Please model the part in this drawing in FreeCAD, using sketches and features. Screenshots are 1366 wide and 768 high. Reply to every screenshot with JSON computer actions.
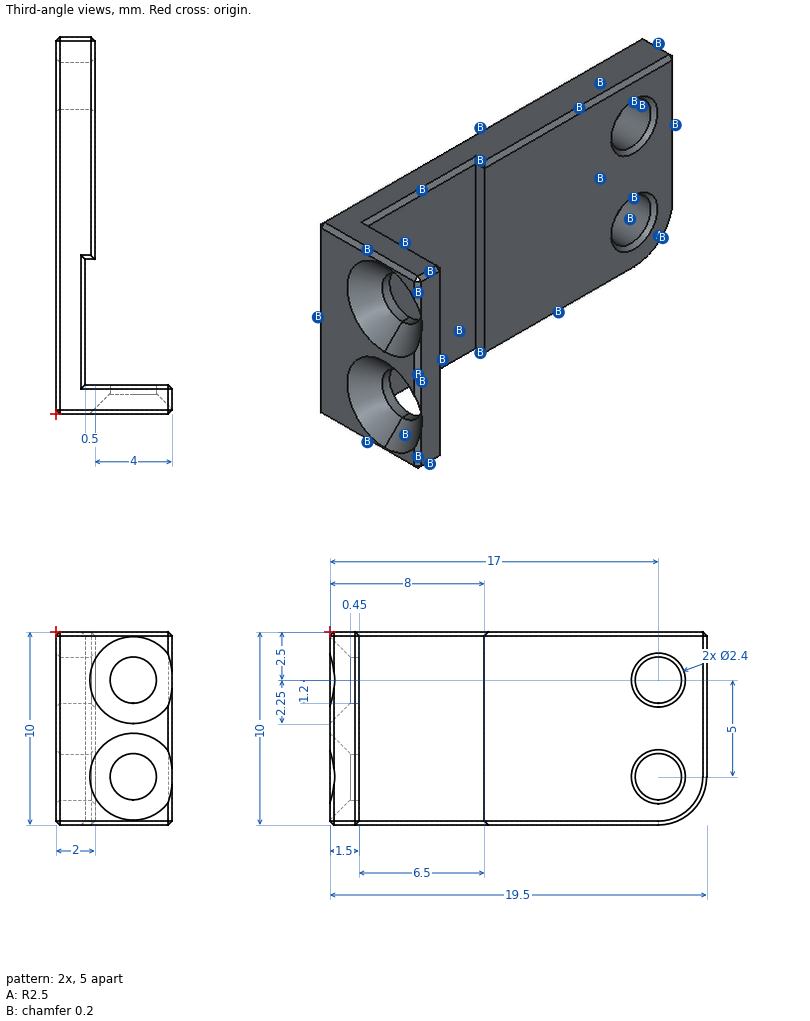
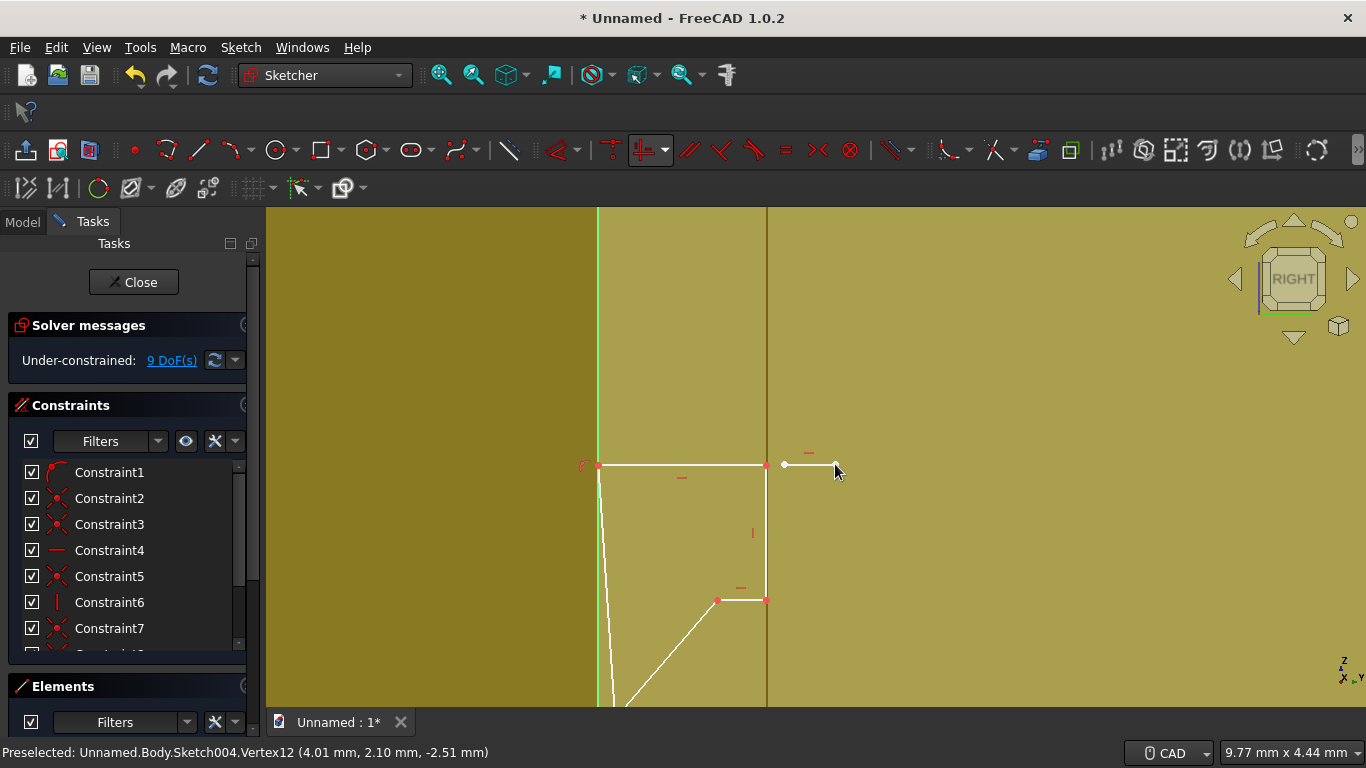
{"action": "left_click", "coordinate": [799, 465]}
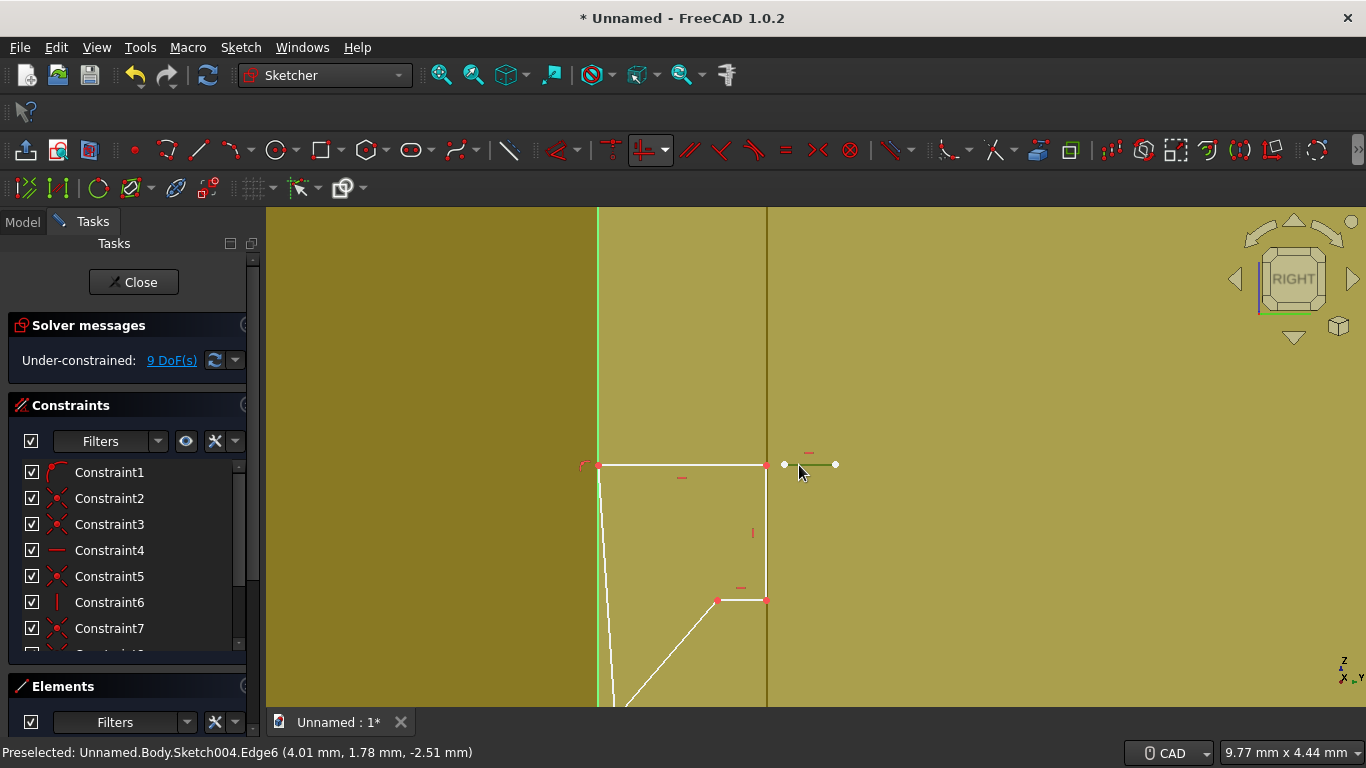
{"action": "left_click", "coordinate": [510, 150]}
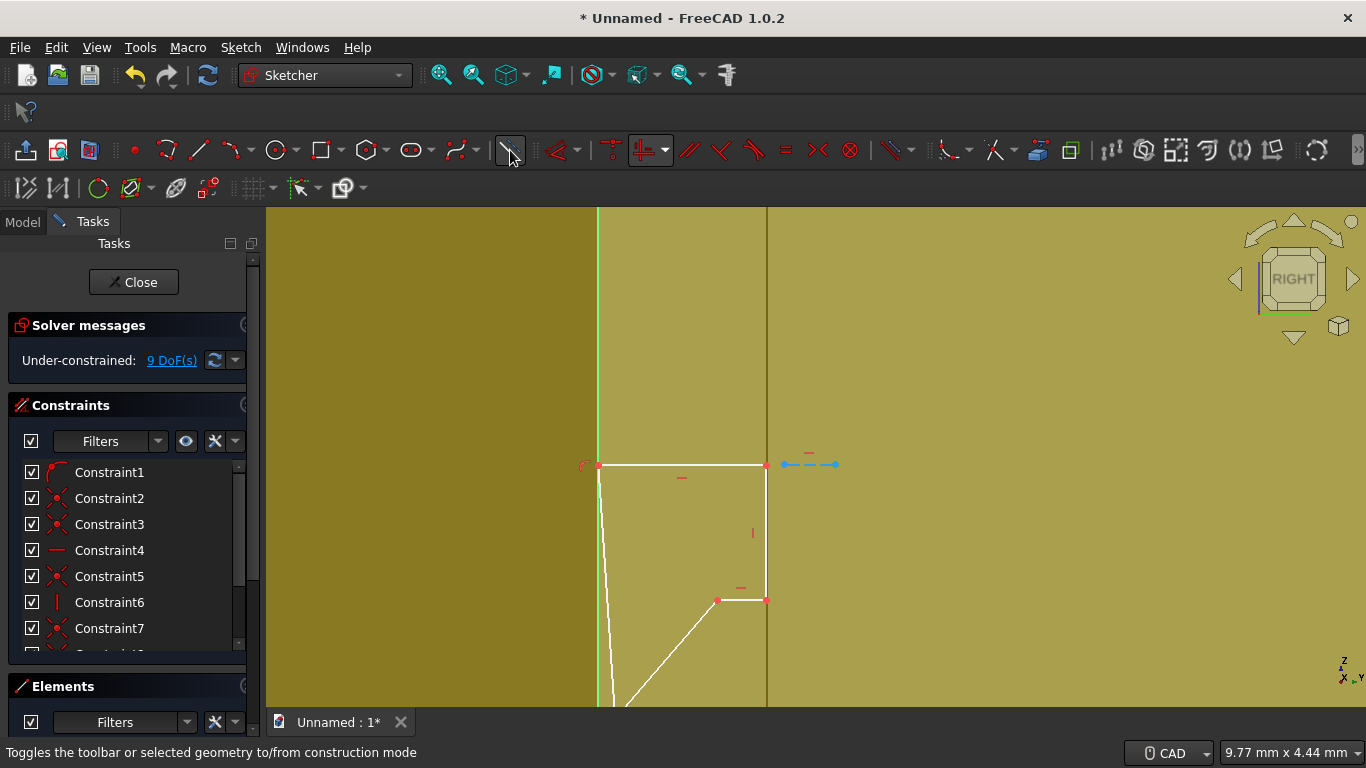
{"action": "left_click", "coordinate": [610, 643]}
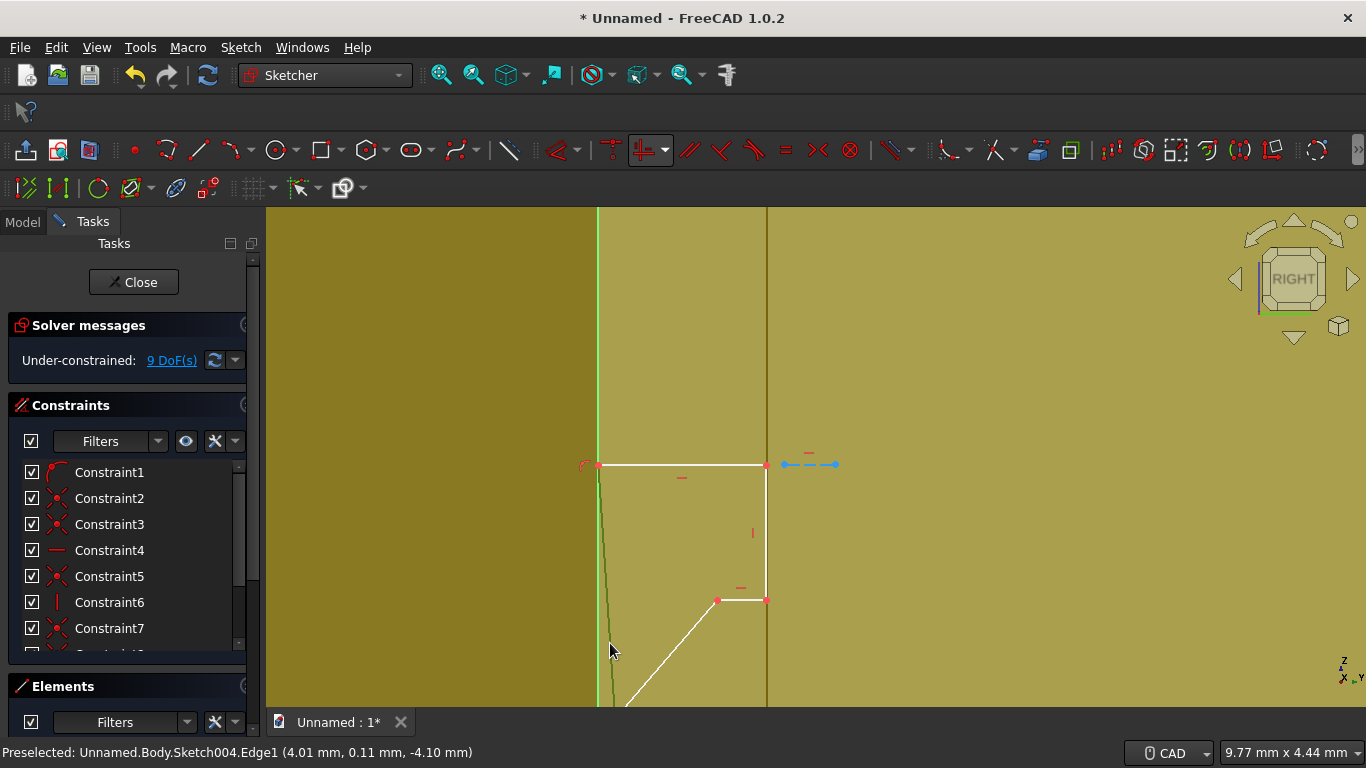
{"action": "left_click", "coordinate": [668, 150]}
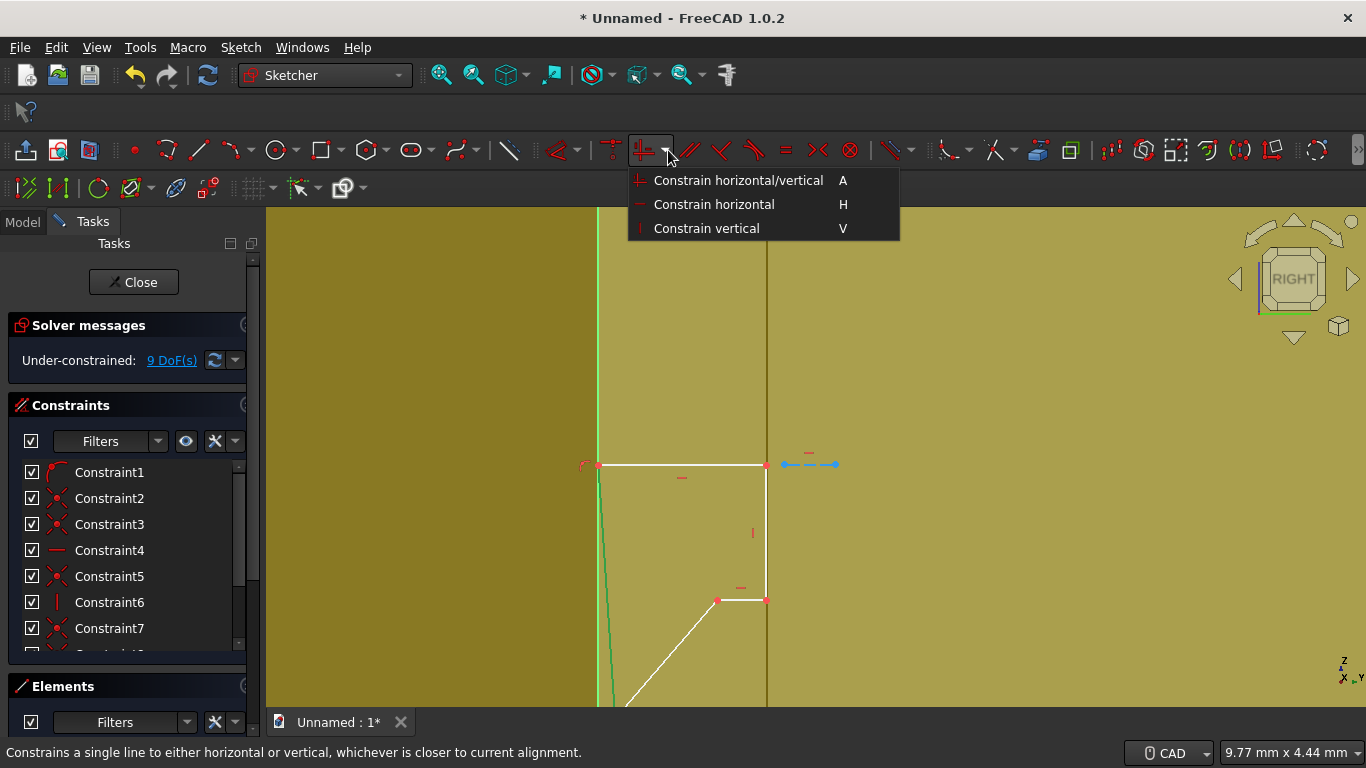
{"action": "left_click", "coordinate": [764, 228]}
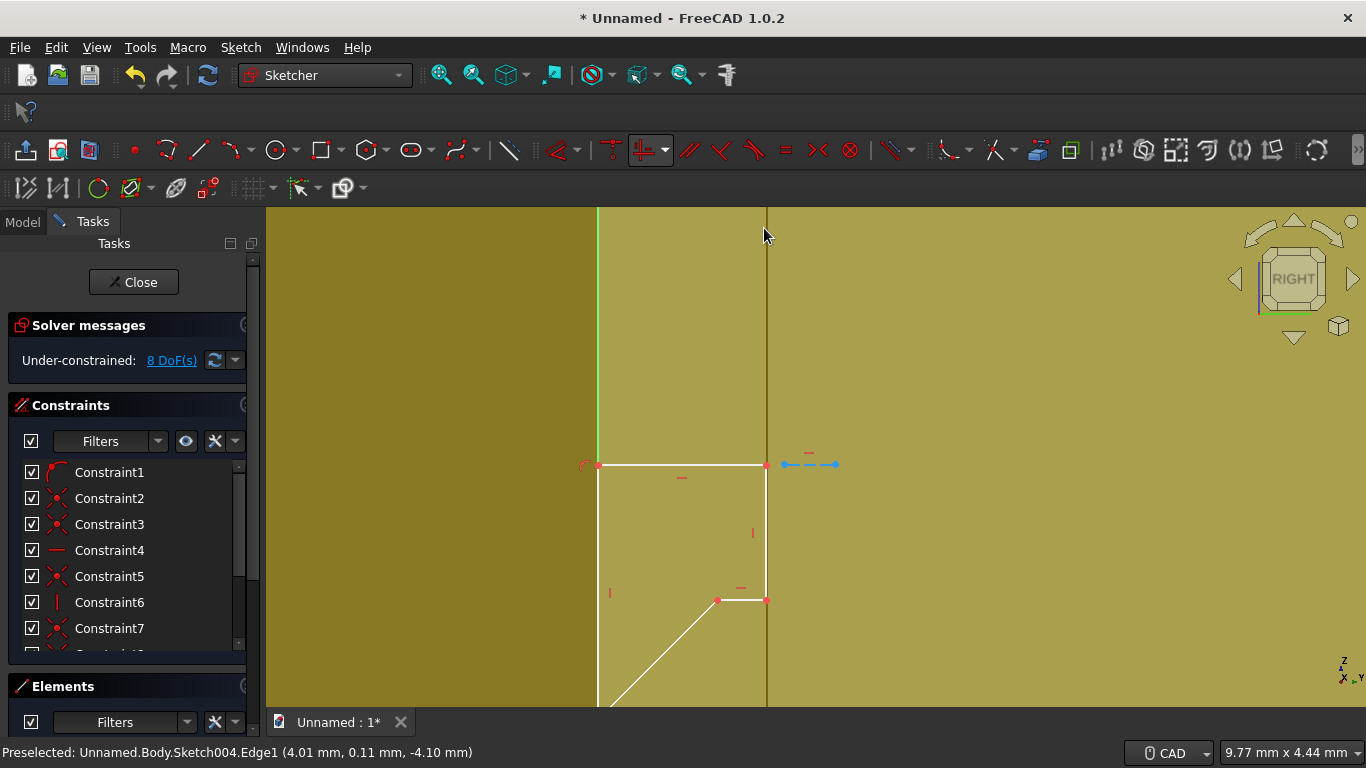
{"action": "left_click", "coordinate": [556, 150]}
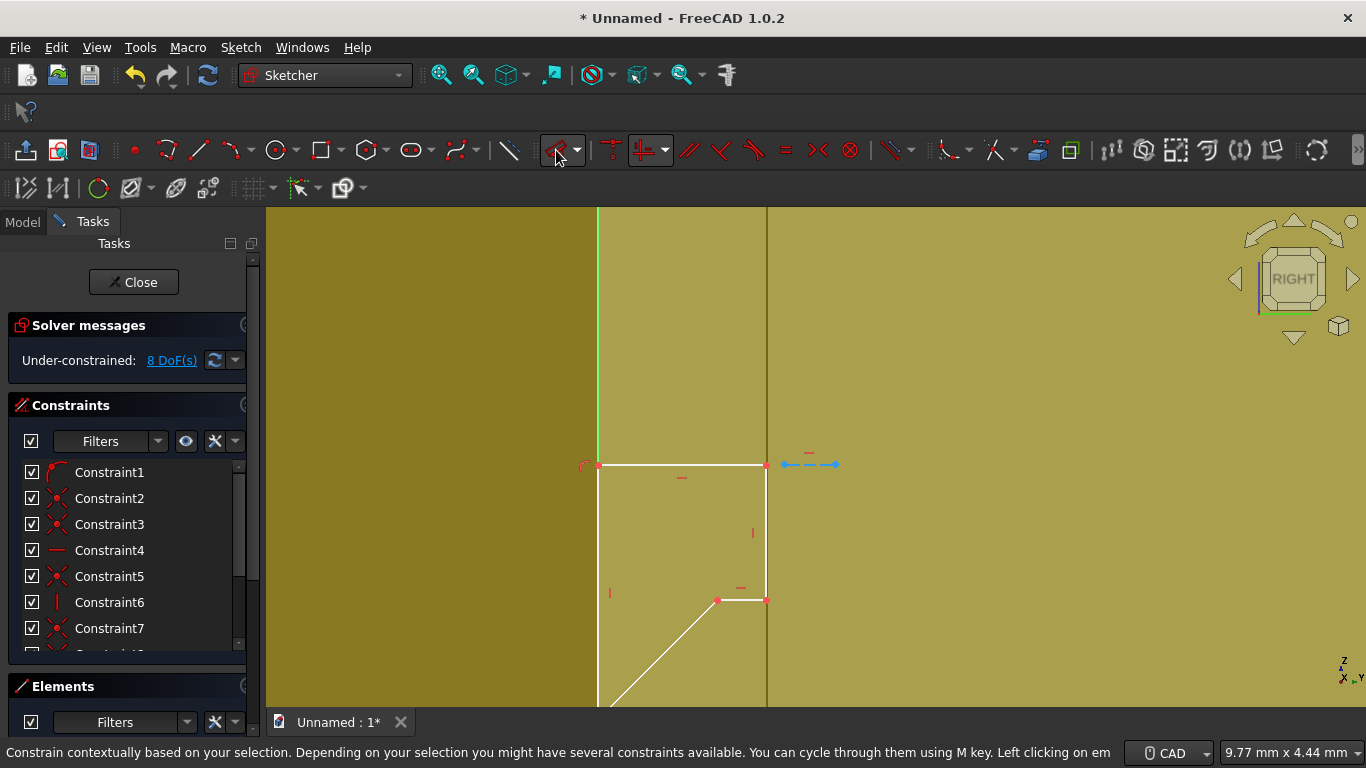
{"action": "left_click", "coordinate": [766, 560]}
{"action": "left_click", "coordinate": [800, 533]}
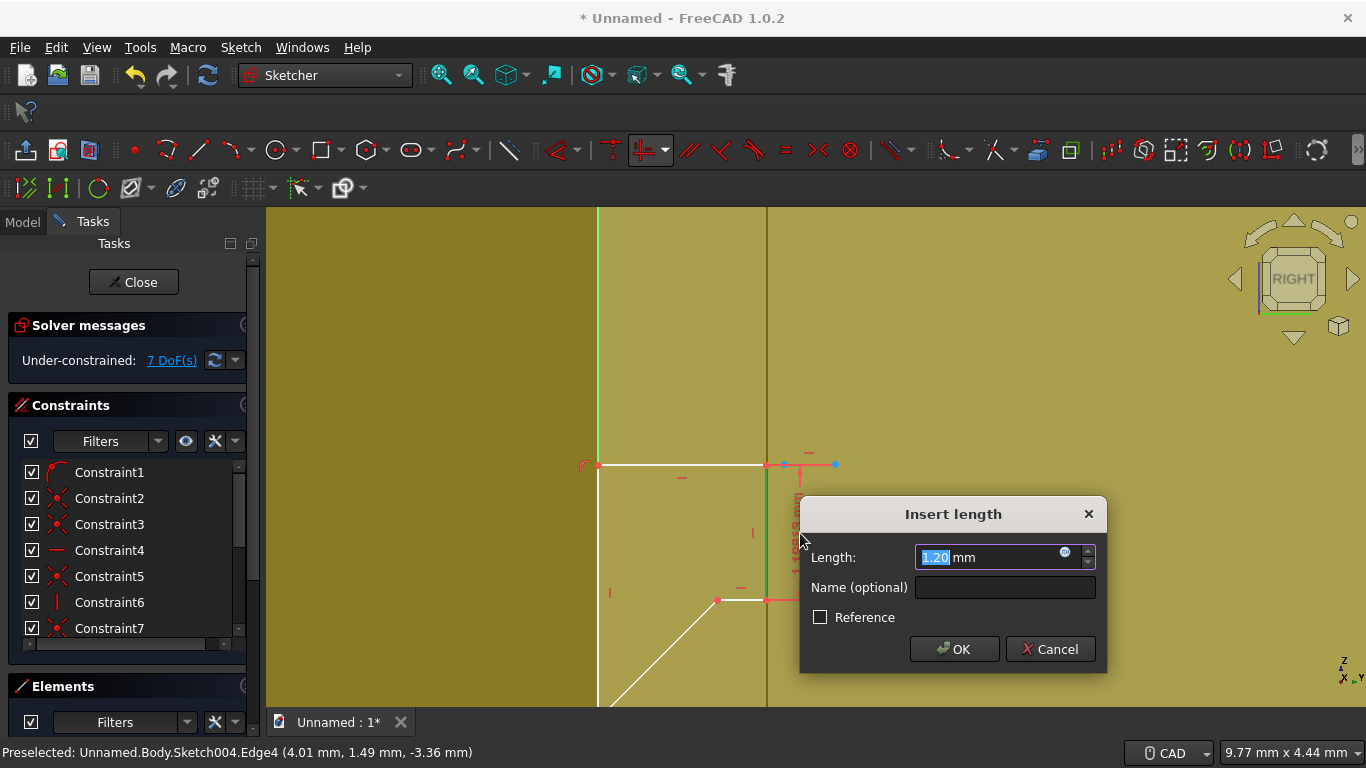
{"action": "type", "text": "1.2"}
{"action": "key", "text": "Return"}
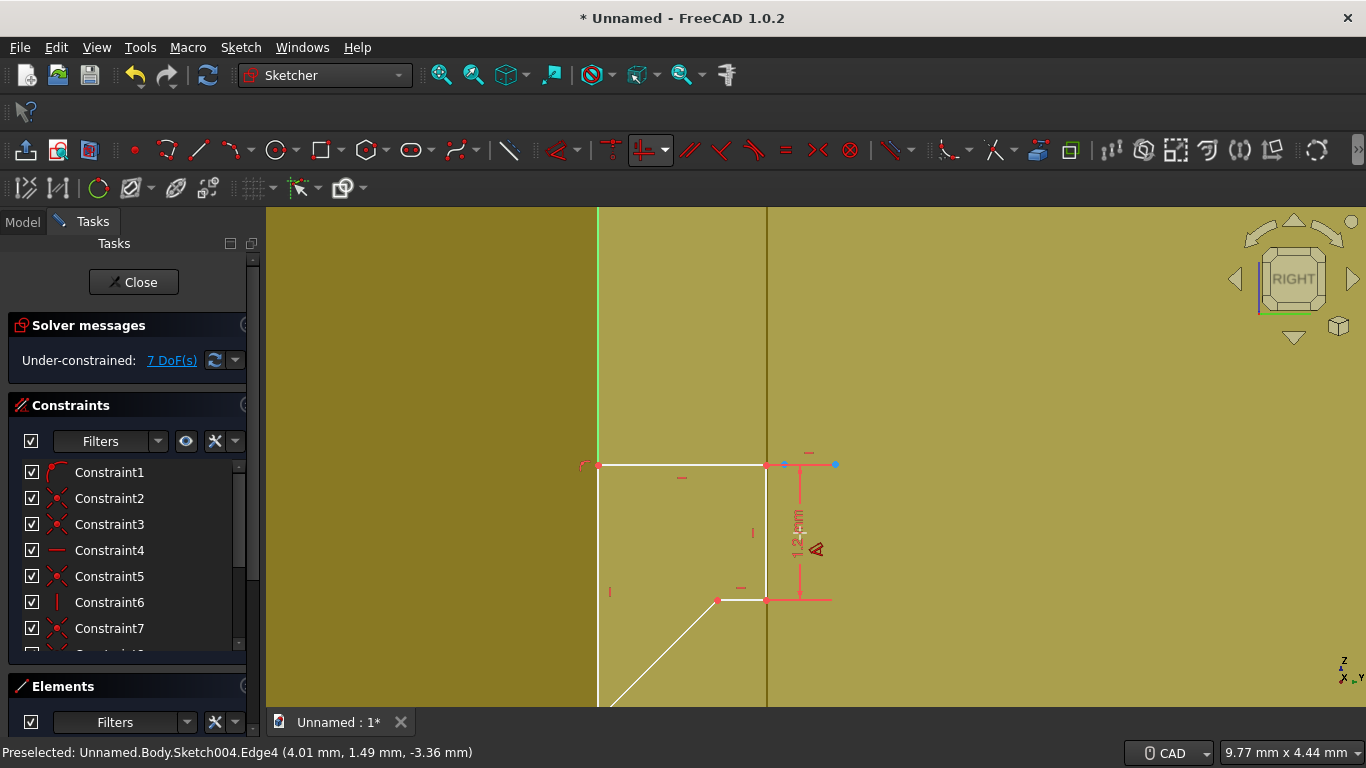
{"action": "left_click", "coordinate": [716, 465]}
{"action": "left_click", "coordinate": [682, 499]}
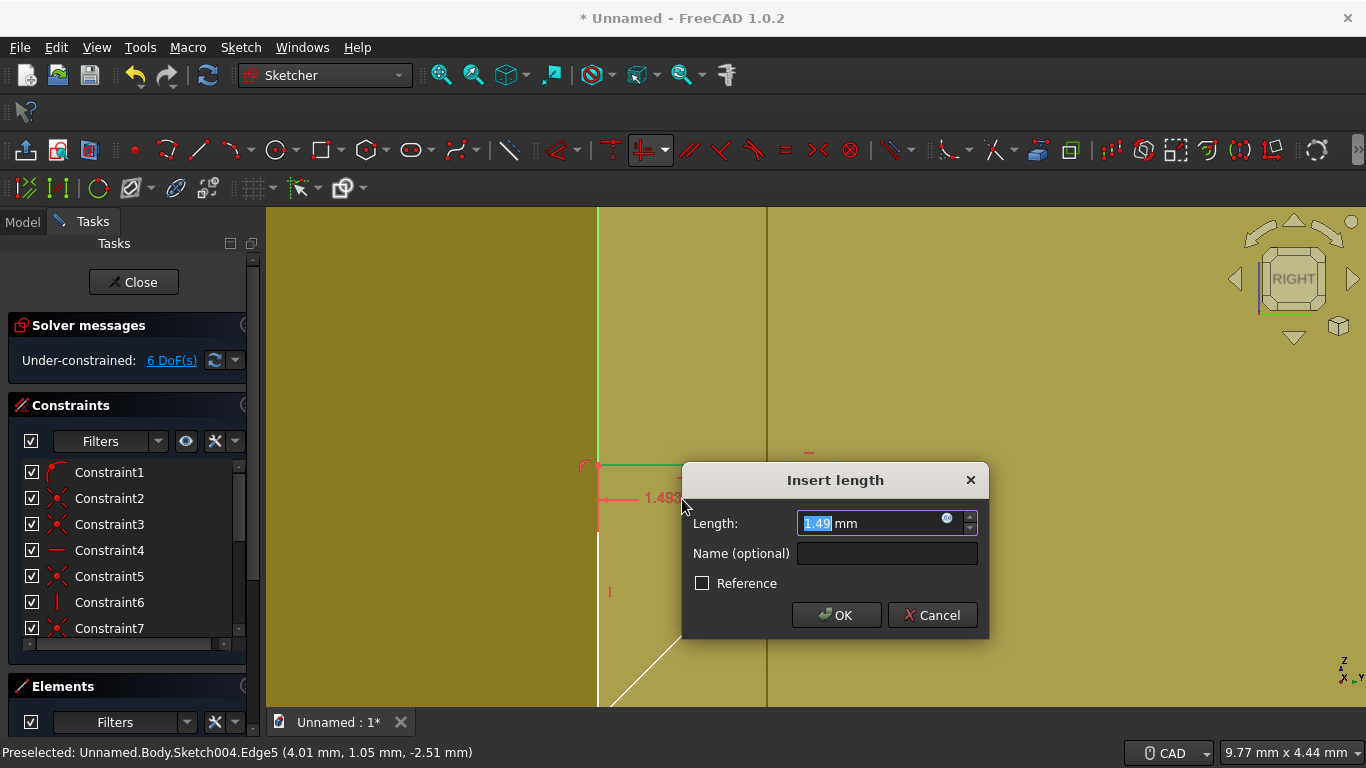
{"action": "type", "text": "1.5"}
{"action": "key", "text": "Return"}